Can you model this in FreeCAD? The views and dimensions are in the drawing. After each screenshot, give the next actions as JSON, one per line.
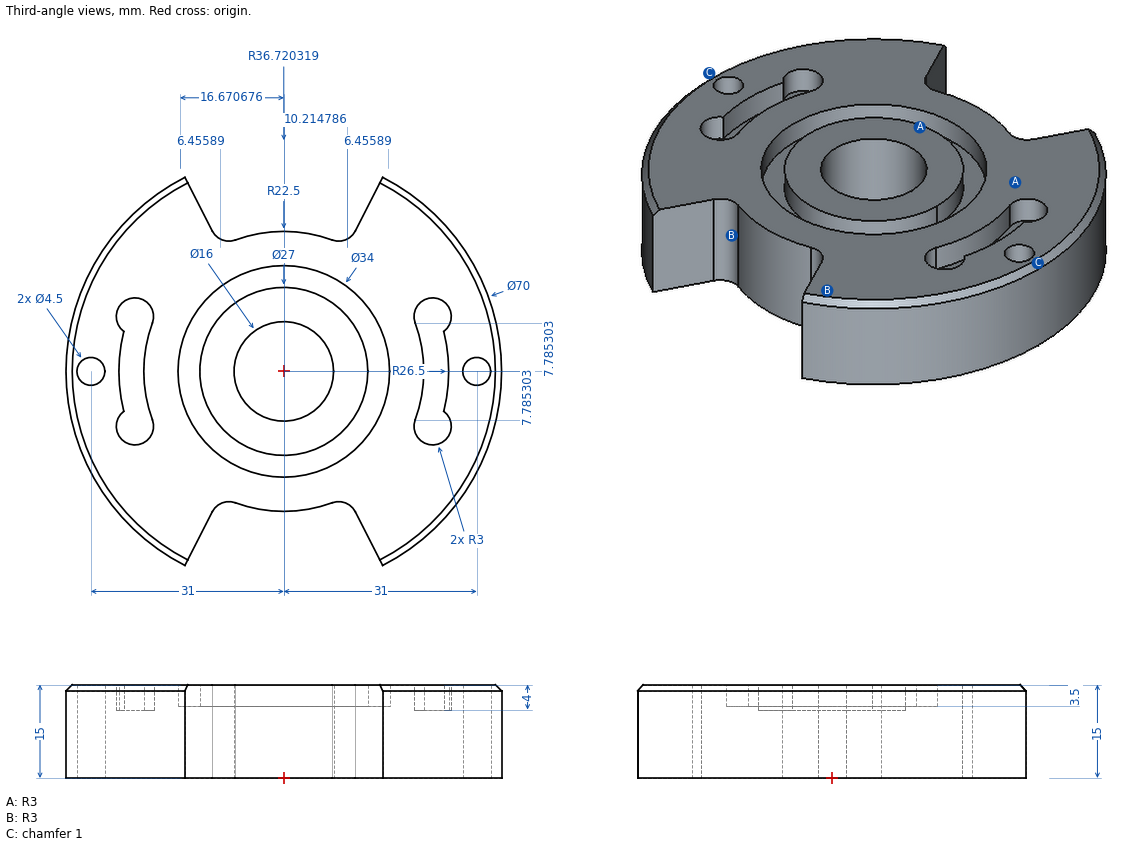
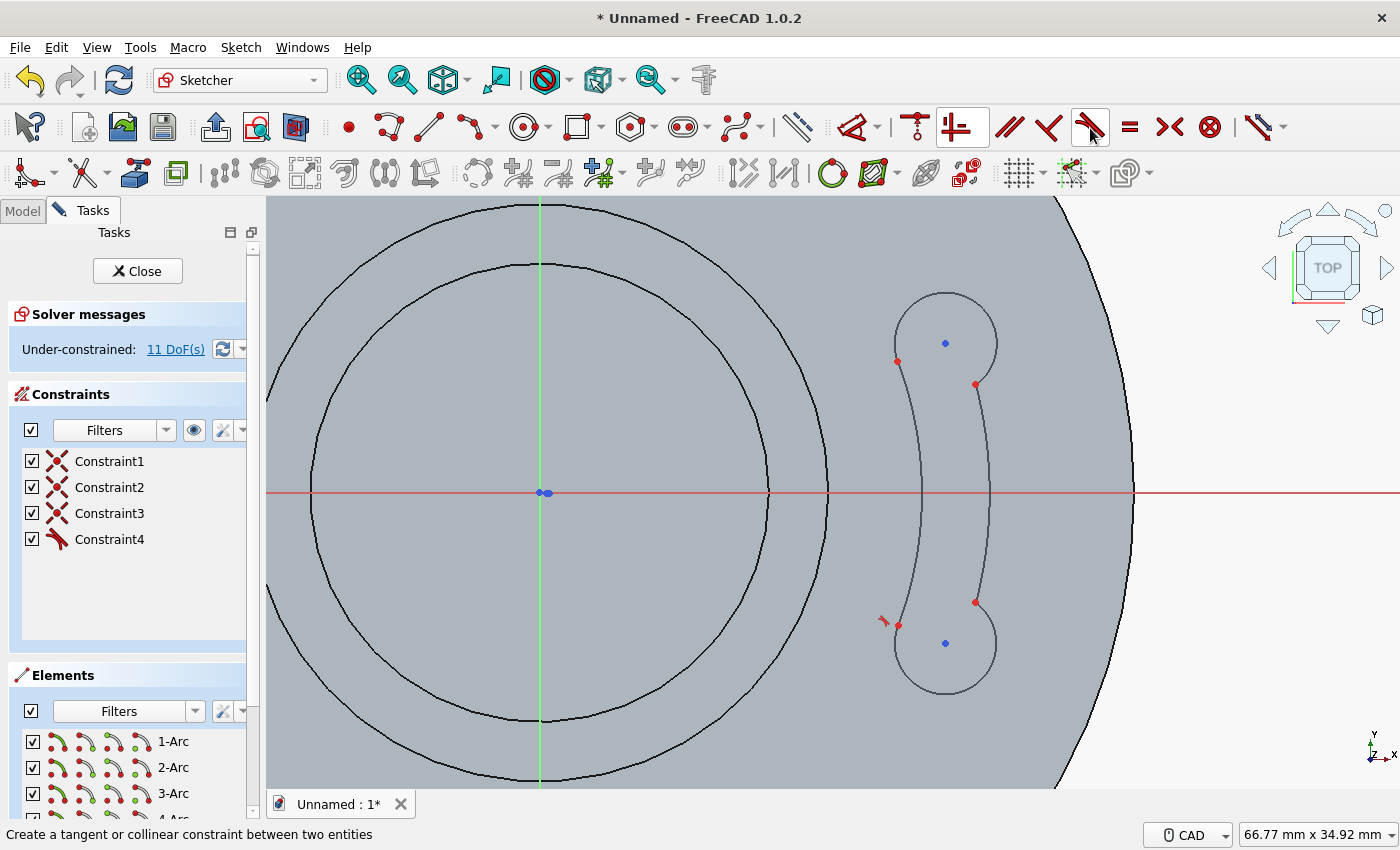
{"action": "left_click", "coordinate": [918, 548]}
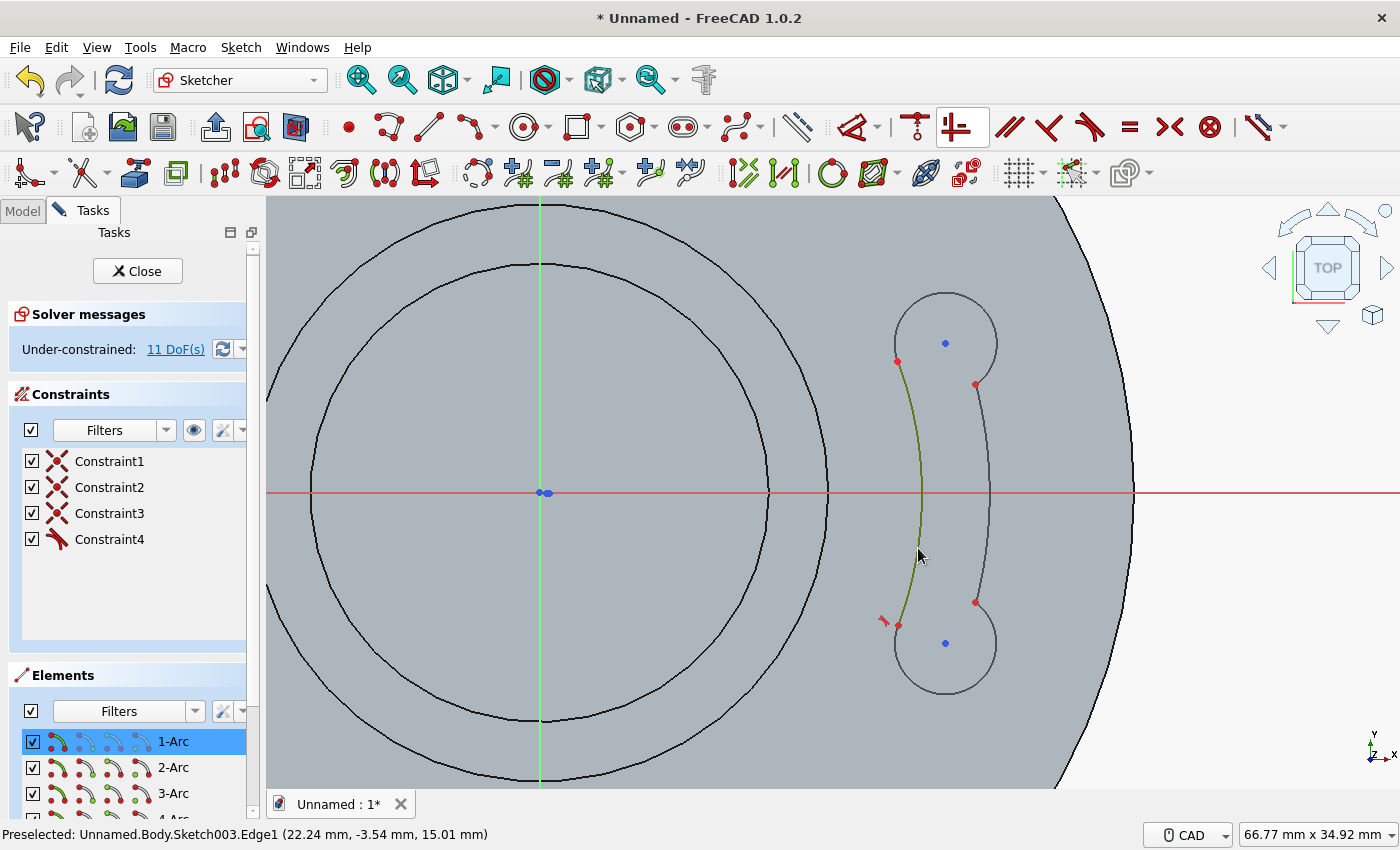
{"action": "left_click", "coordinate": [993, 324]}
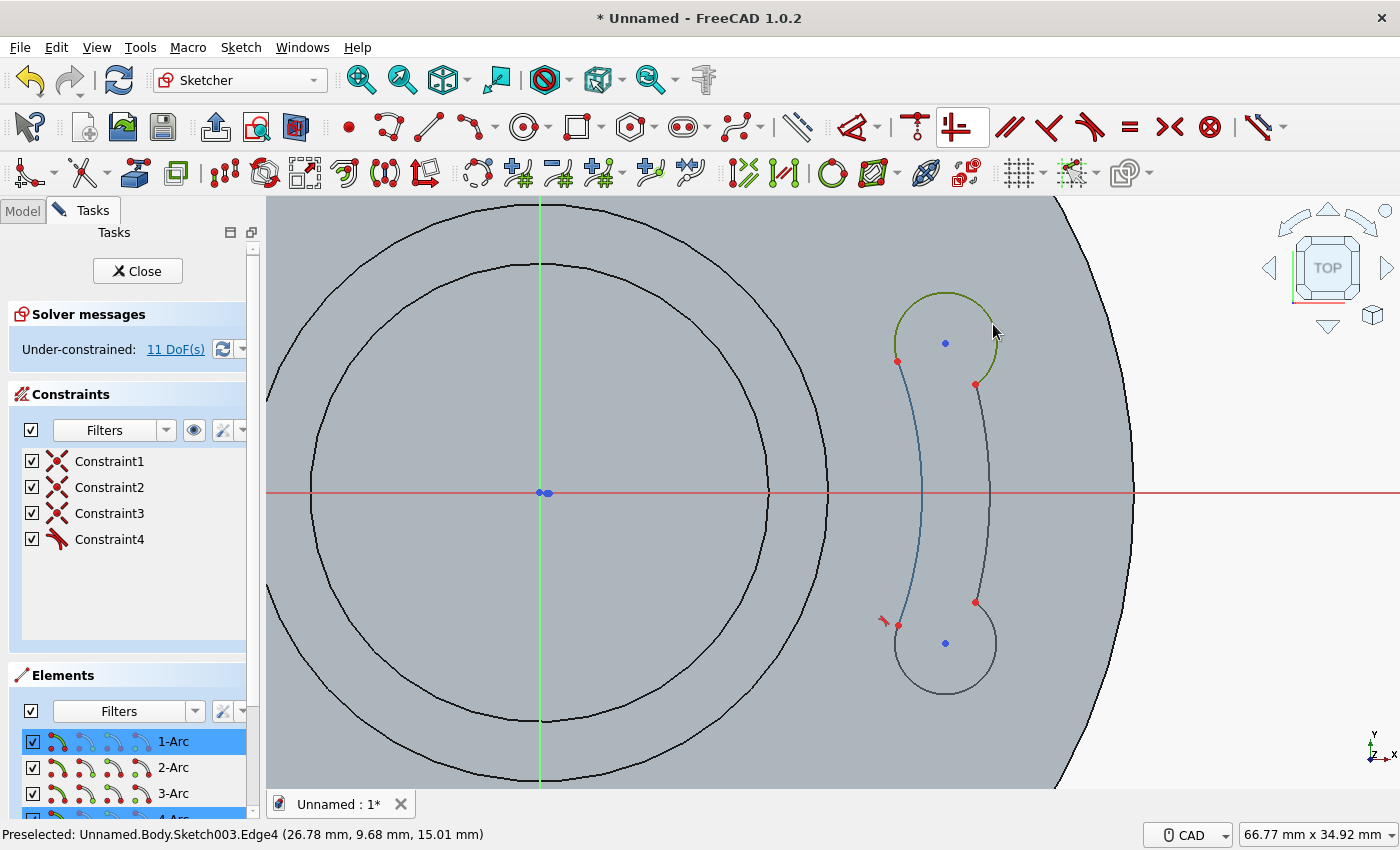
{"action": "key", "text": "t"}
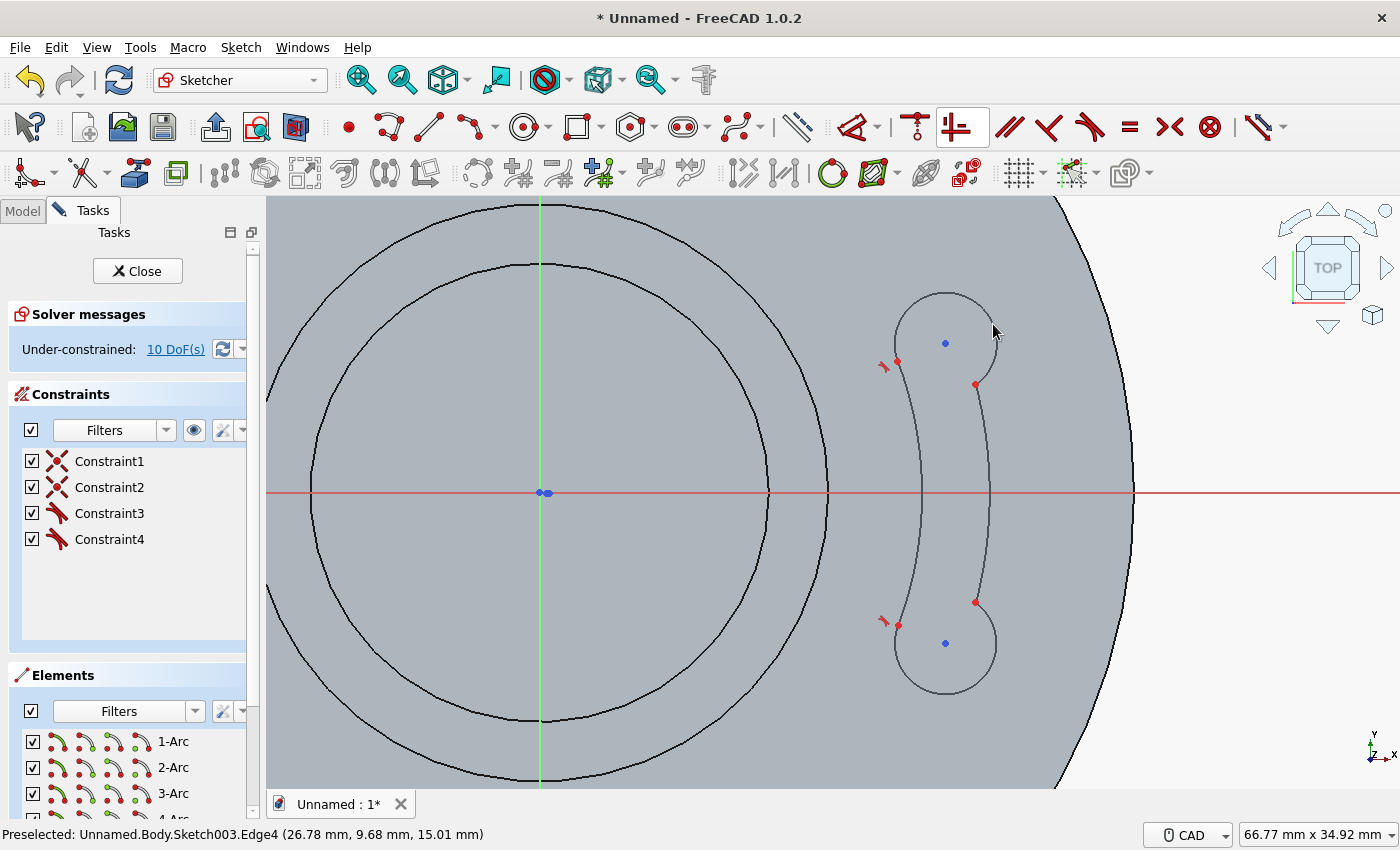
{"action": "left_click", "coordinate": [918, 548]}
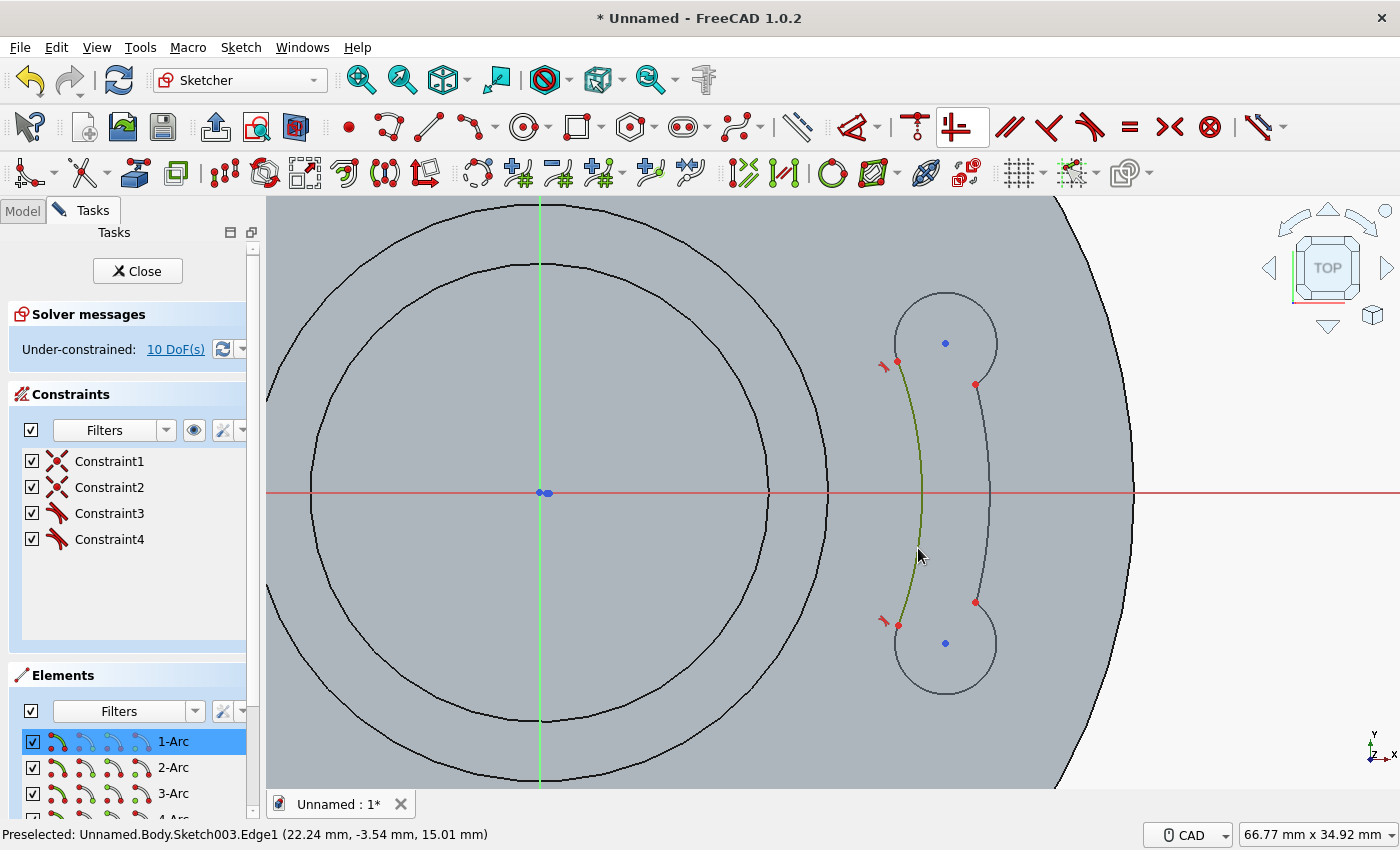
{"action": "left_click", "coordinate": [987, 538]}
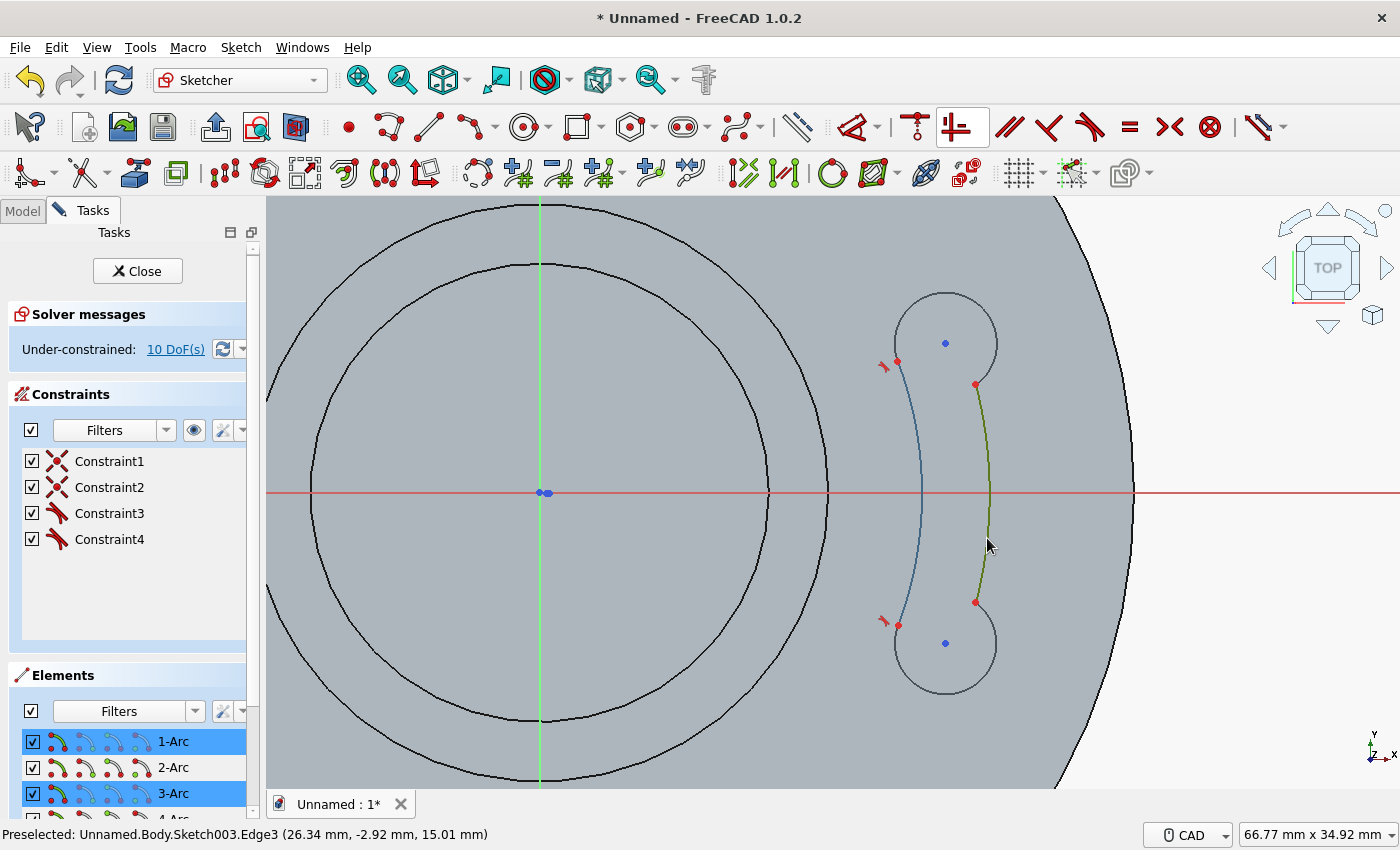
{"action": "left_click", "coordinate": [916, 128]}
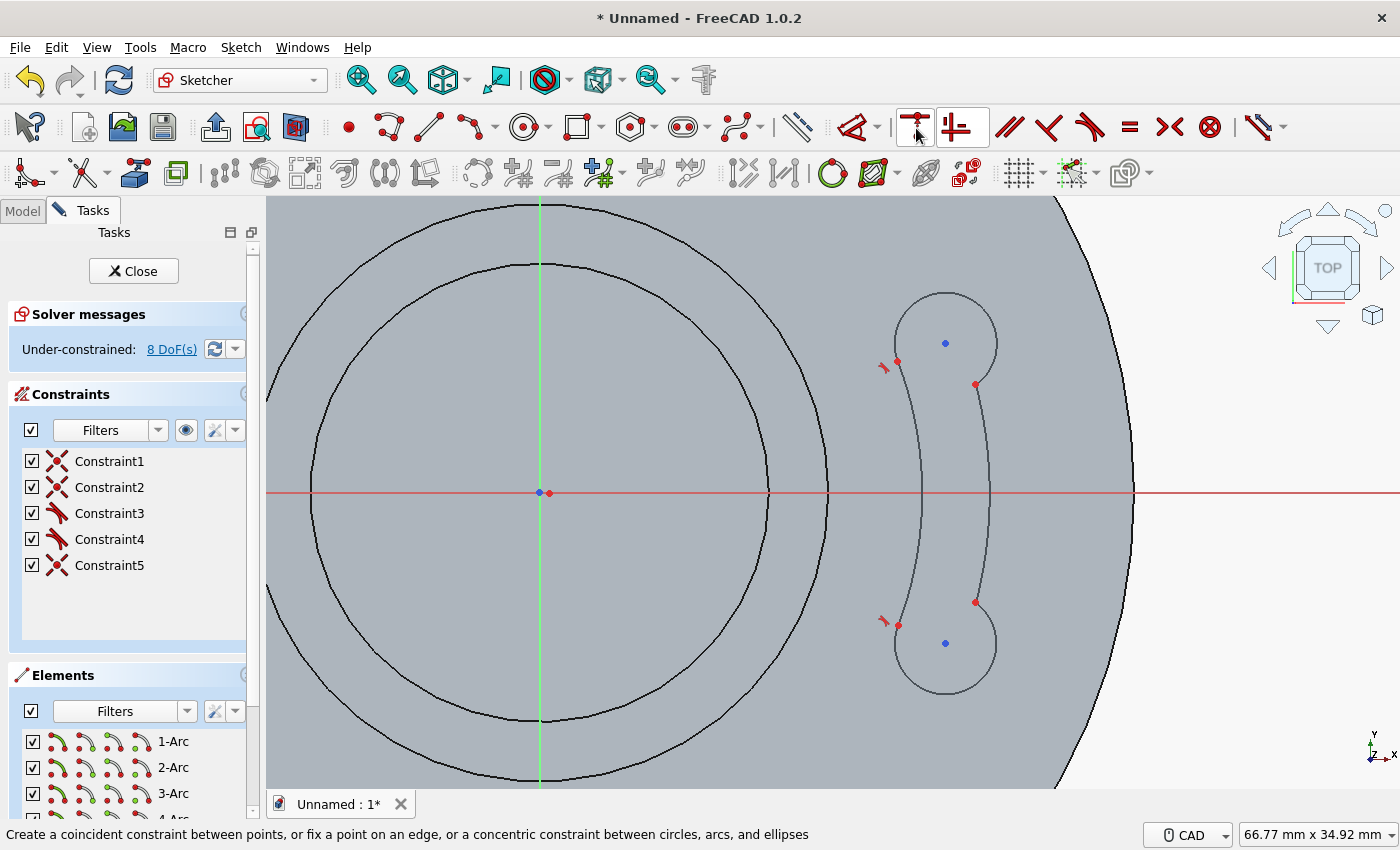
{"action": "left_click_drag", "start_coordinate": [530, 483], "coordinate": [560, 504]}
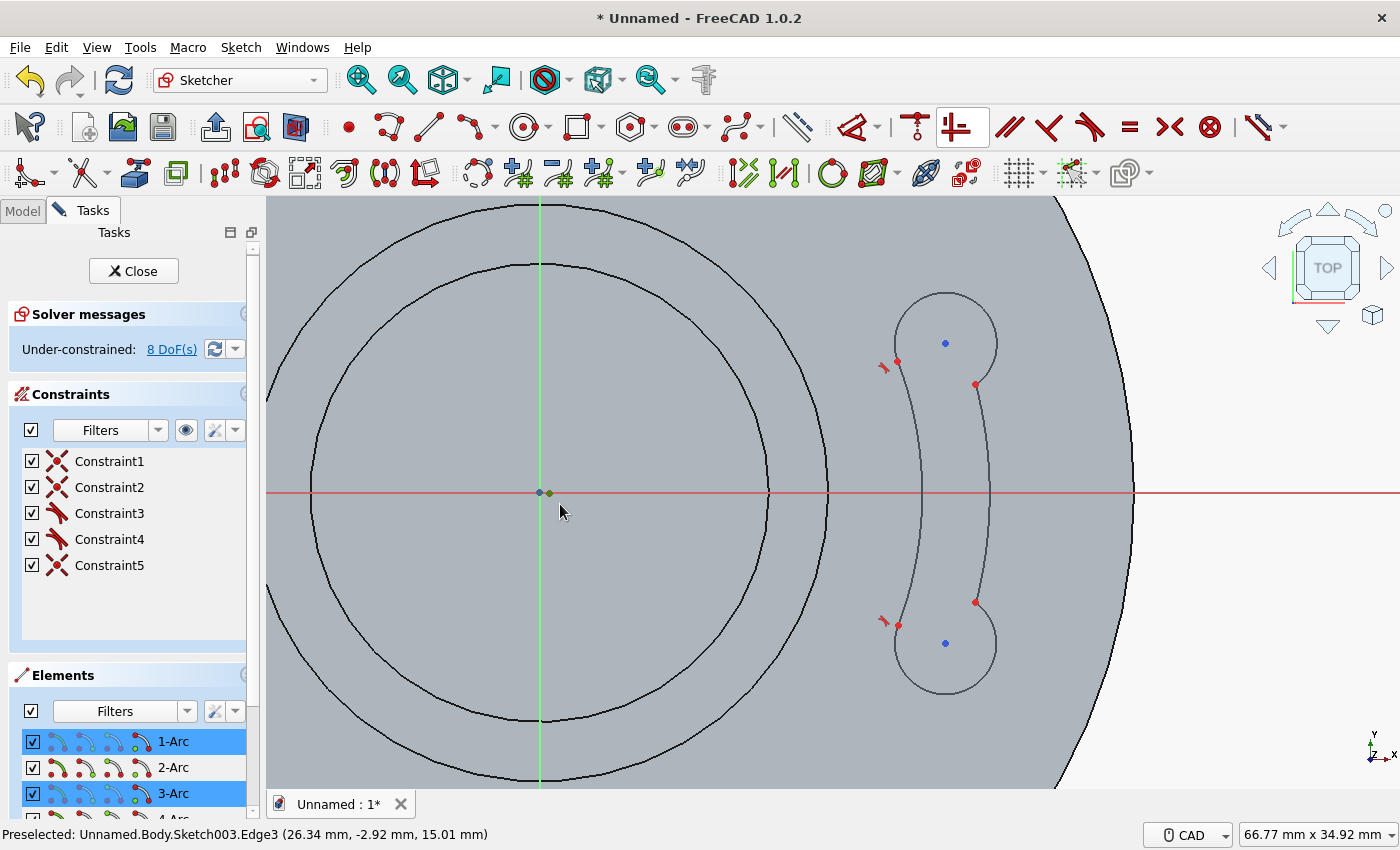
{"action": "left_click", "coordinate": [916, 128]}